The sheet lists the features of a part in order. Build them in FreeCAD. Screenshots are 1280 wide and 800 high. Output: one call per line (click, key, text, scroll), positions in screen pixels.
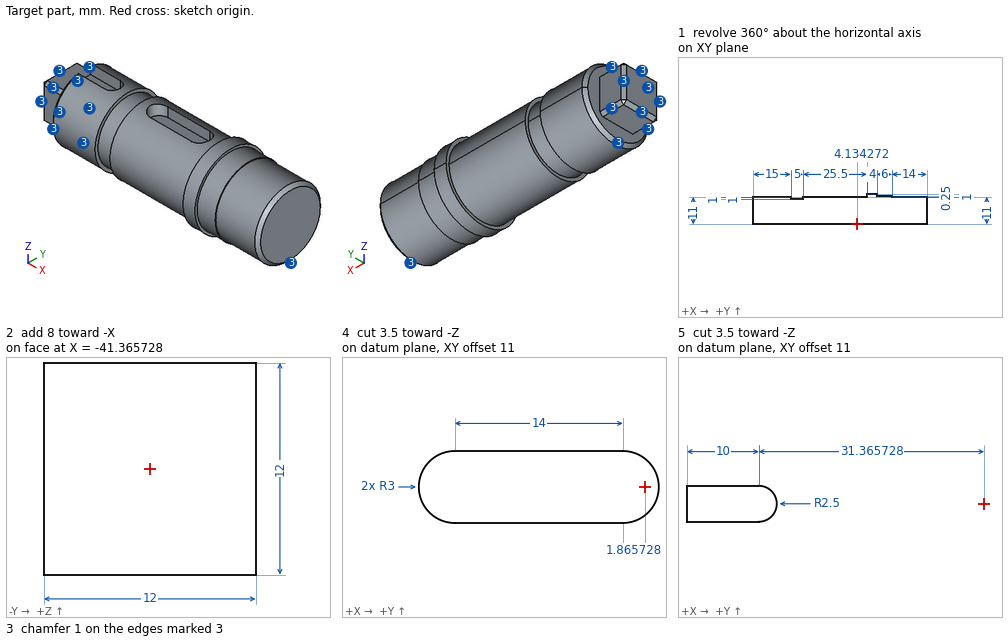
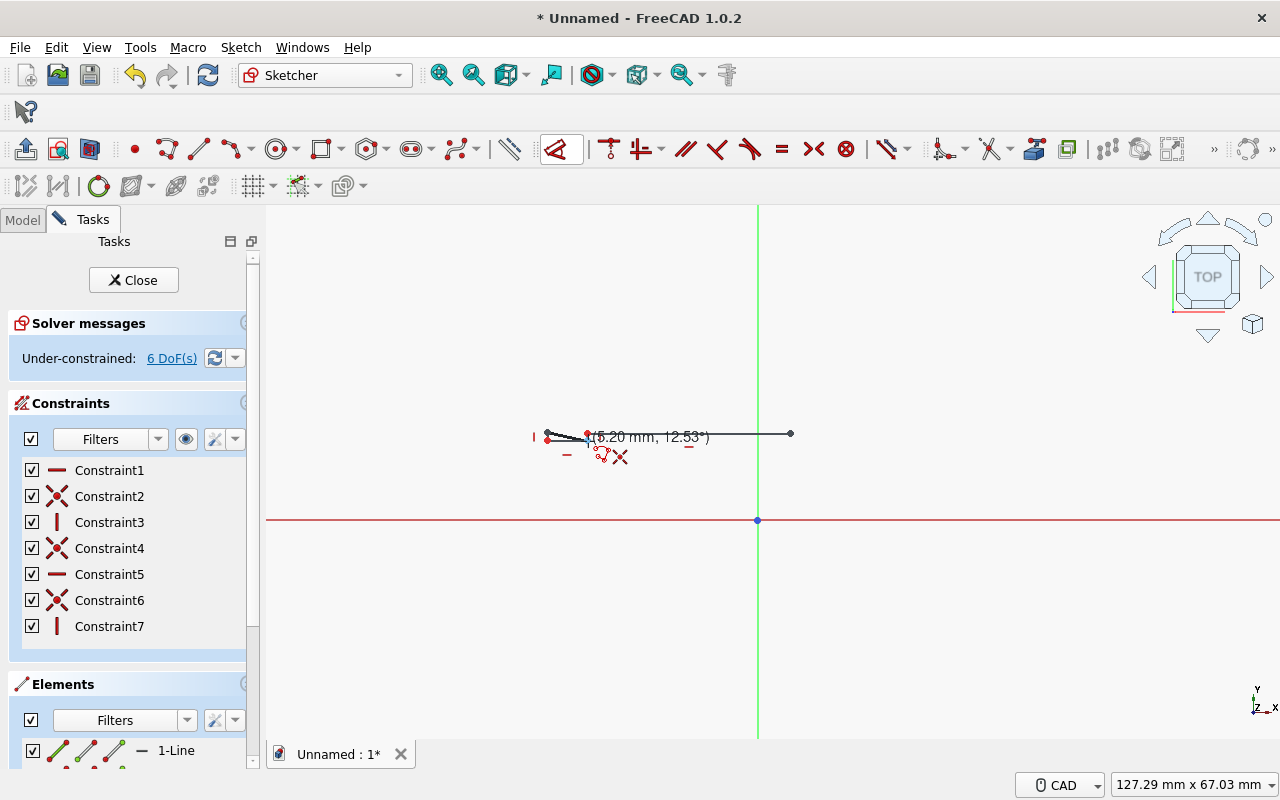
click(428, 432)
click(428, 520)
click(982, 511)
click(982, 432)
click(870, 432)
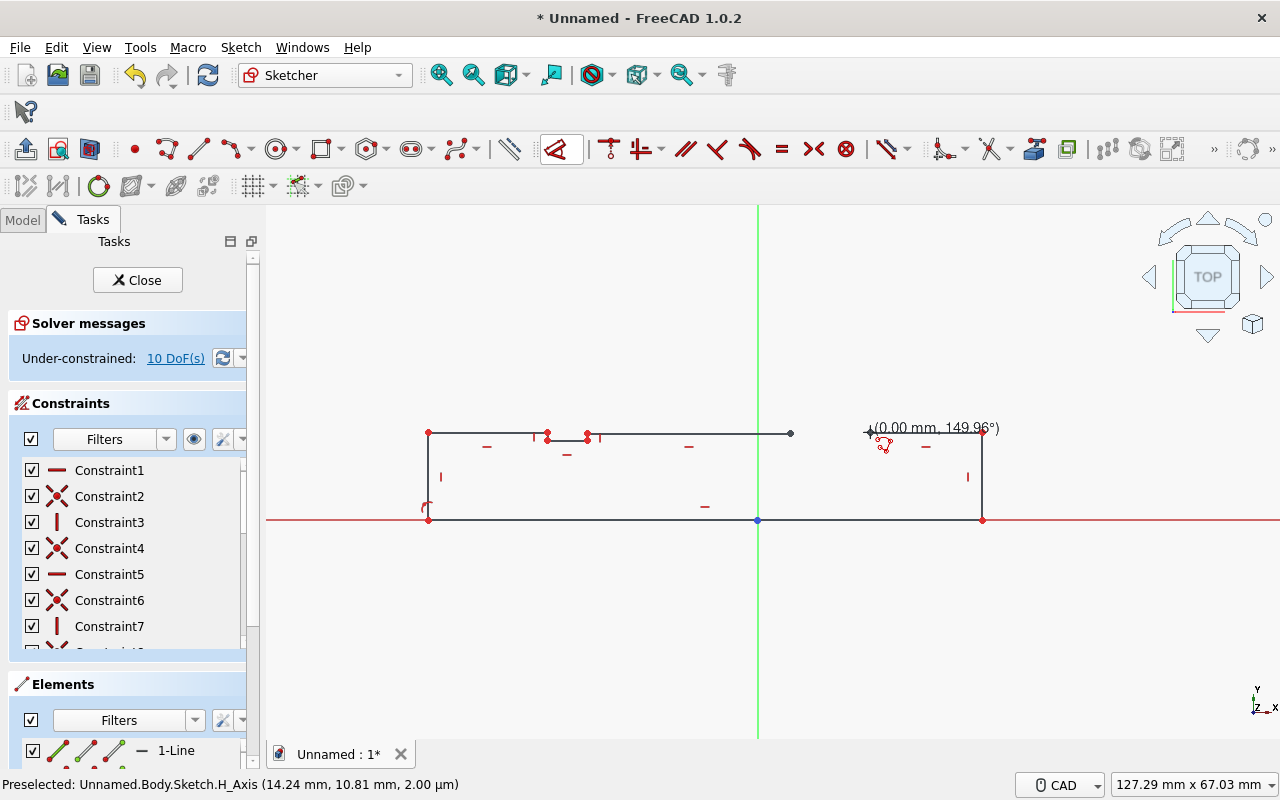
scroll(870, 430, up, 11)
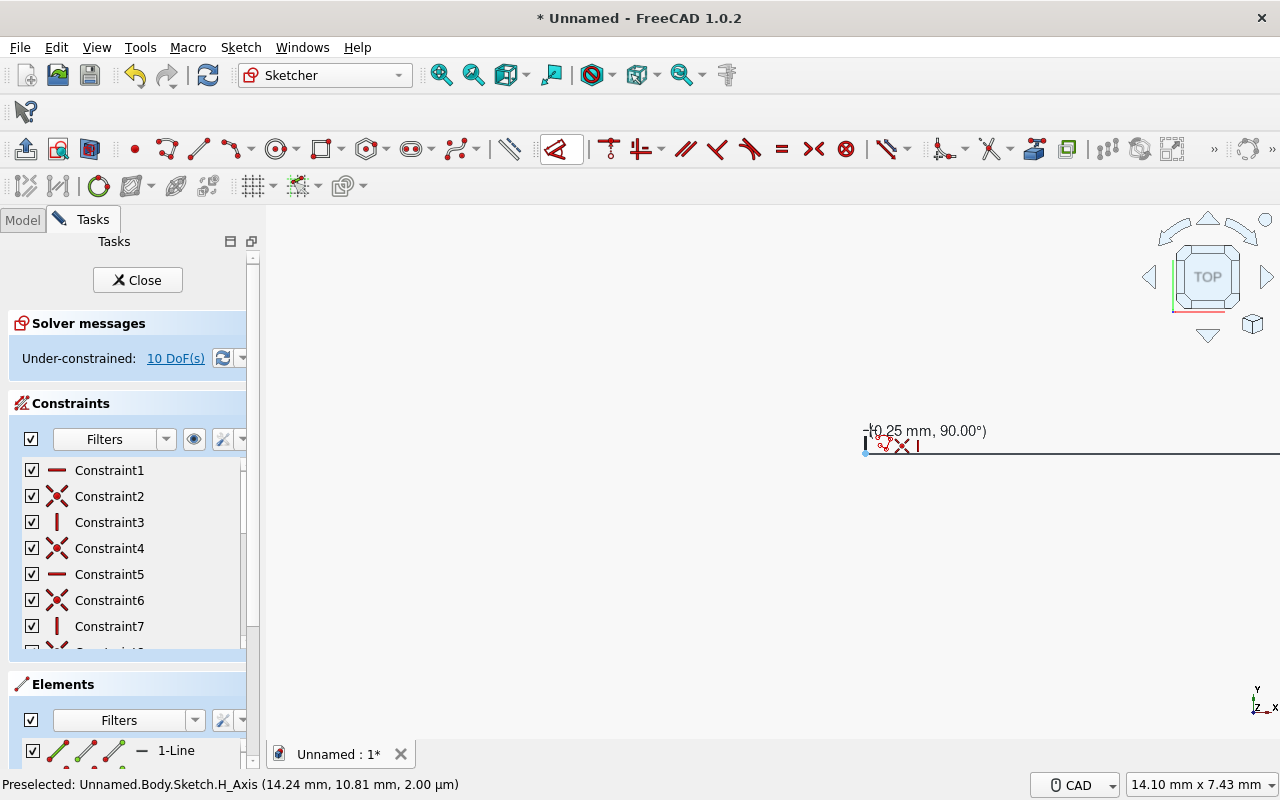
click(865, 431)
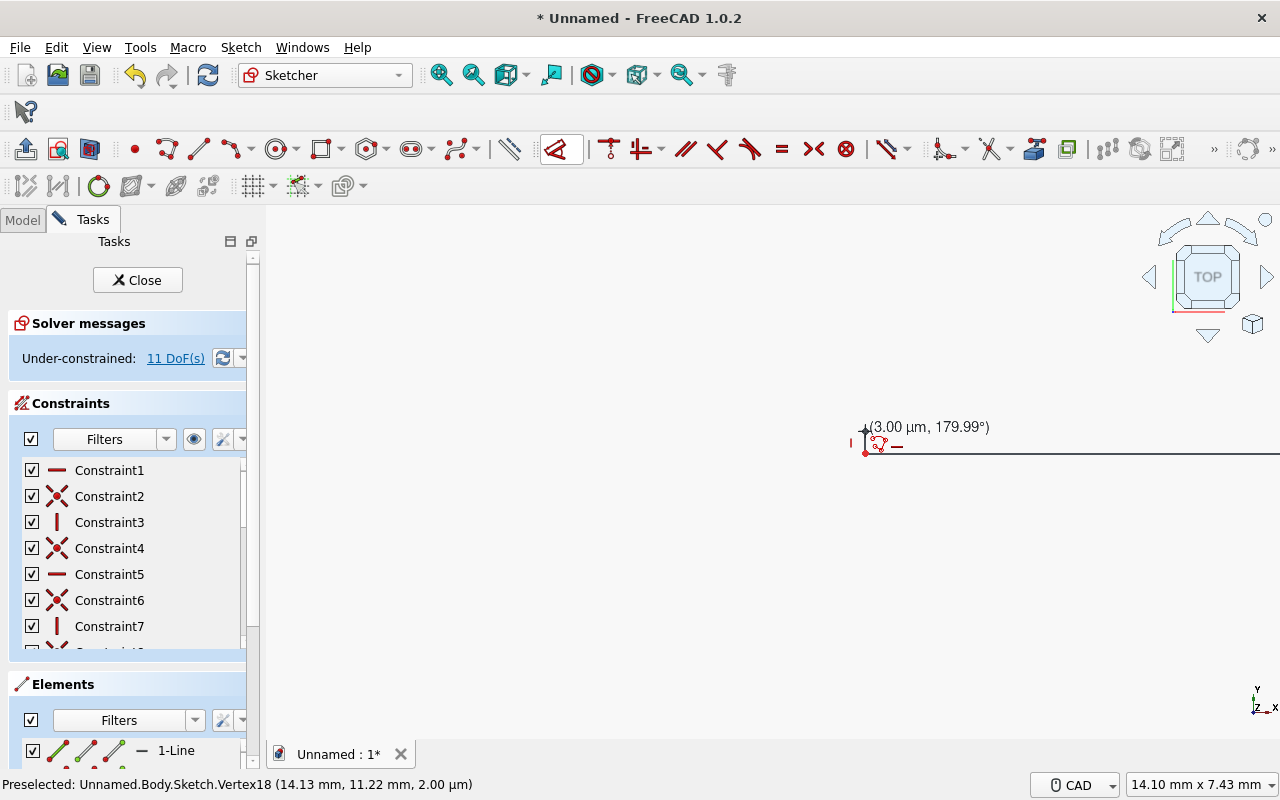
scroll(870, 430, down, 11)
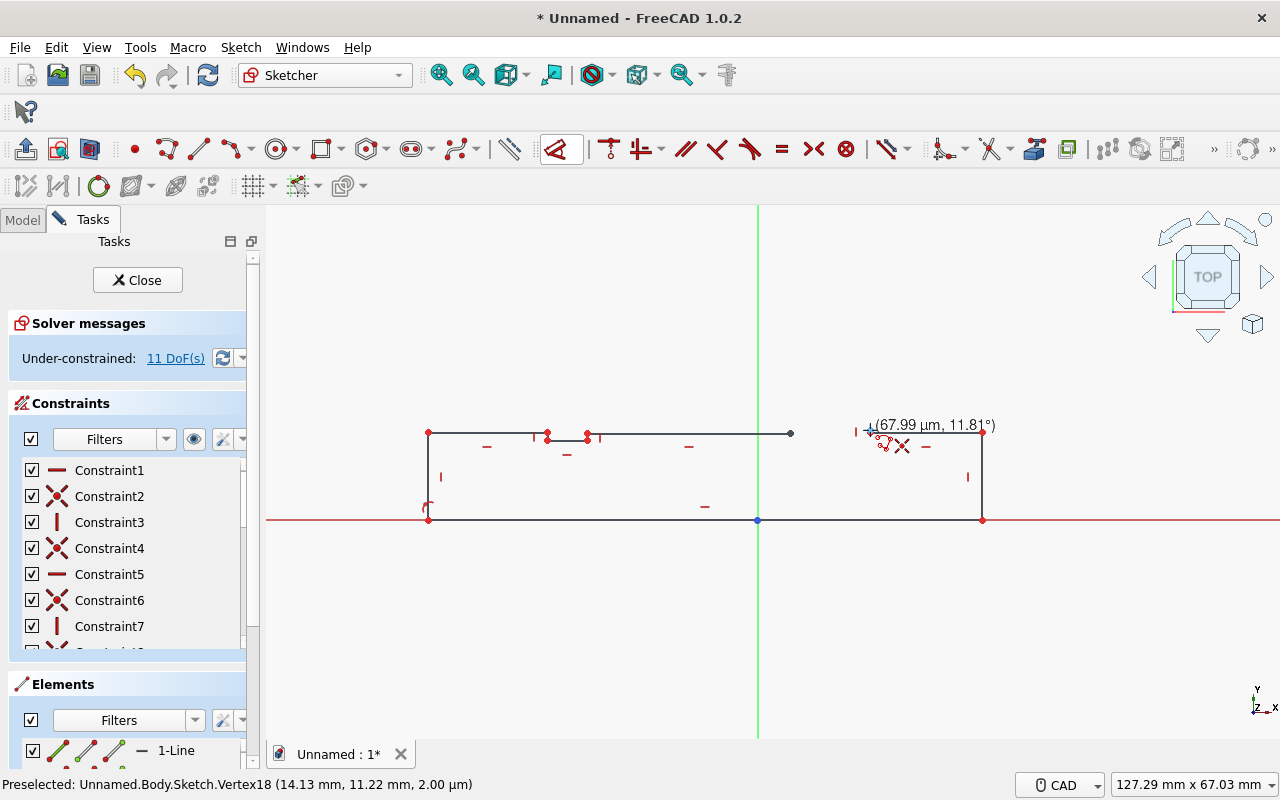
click(822, 430)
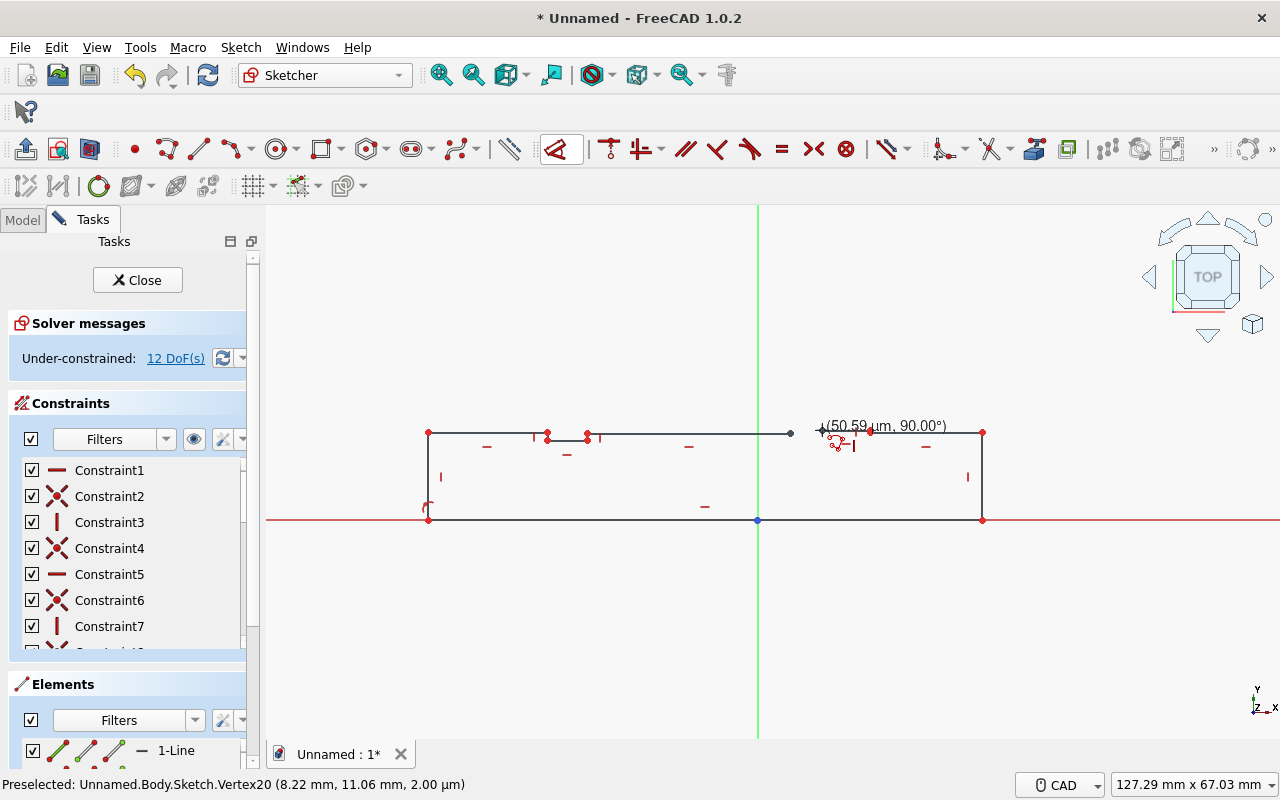
scroll(822, 425, up, 5)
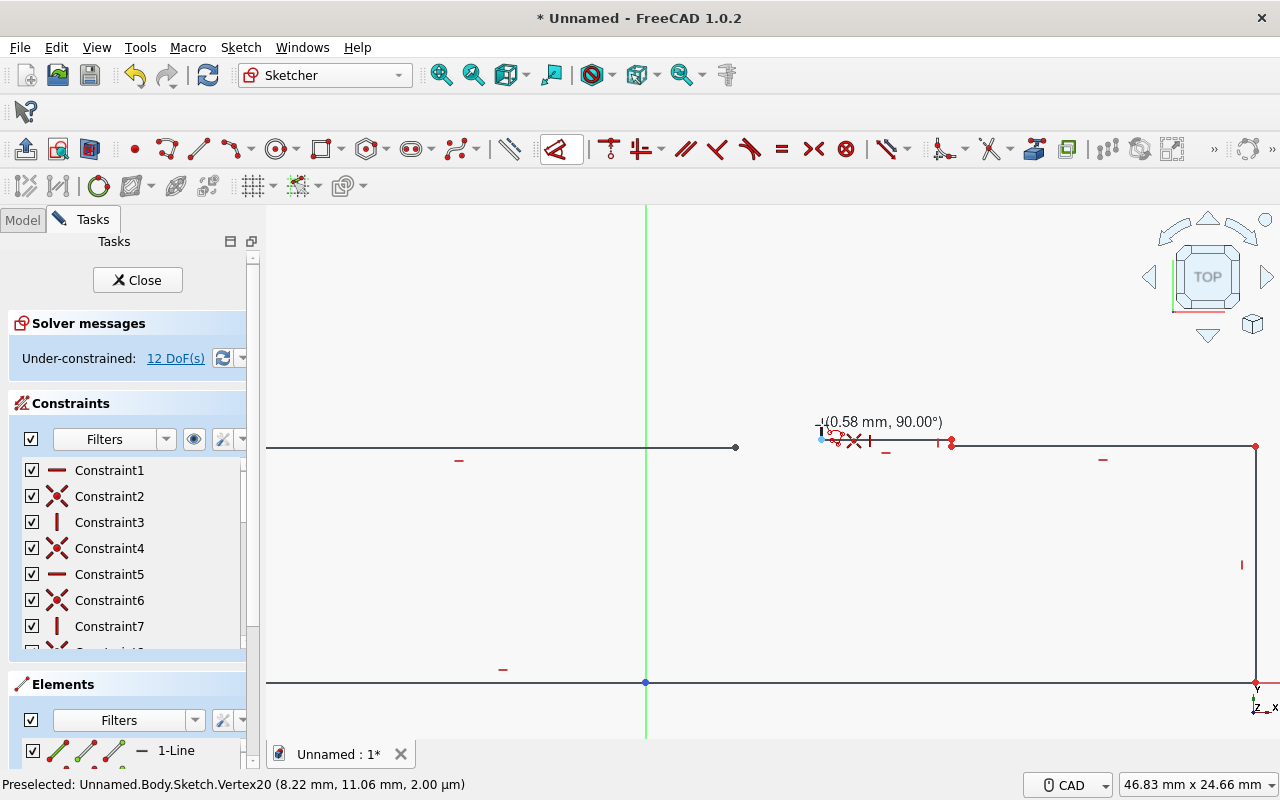
click(821, 423)
click(735, 423)
click(736, 448)
key(Escape)
key(Escape)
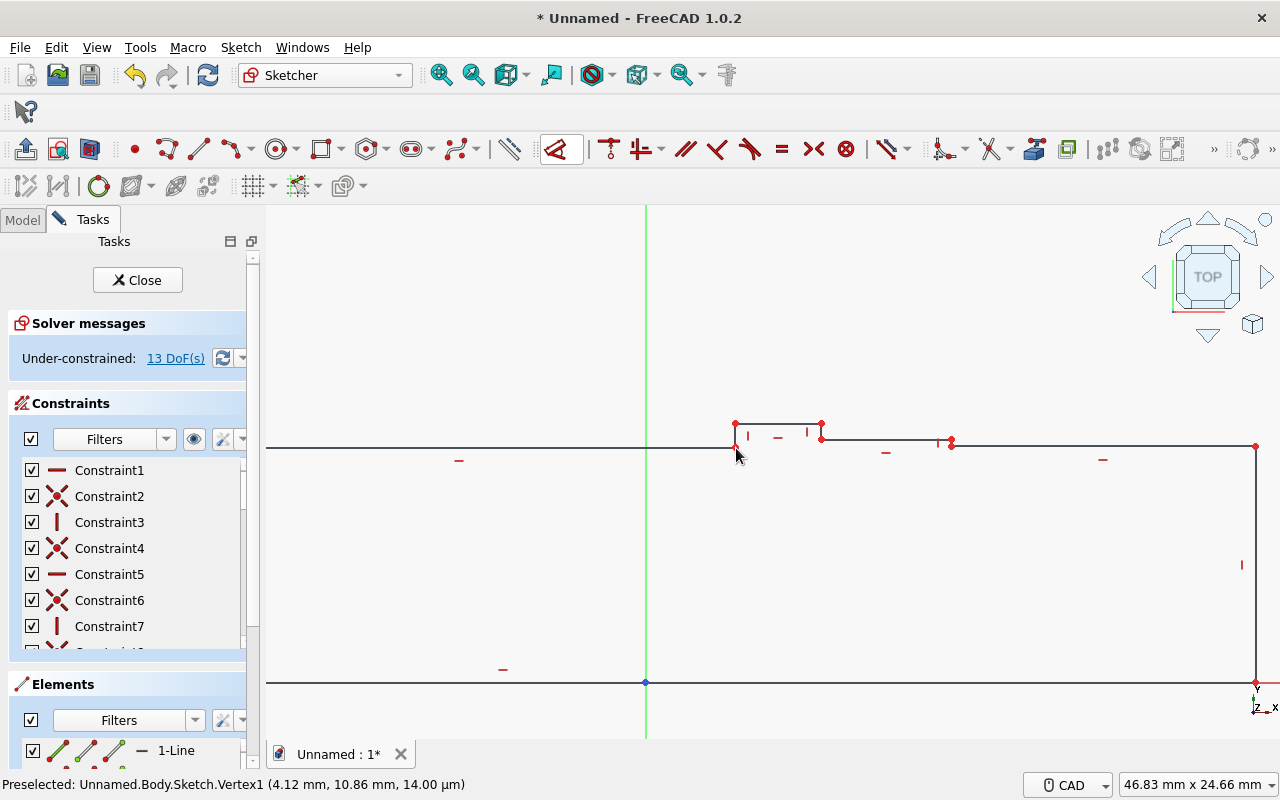
click(556, 150)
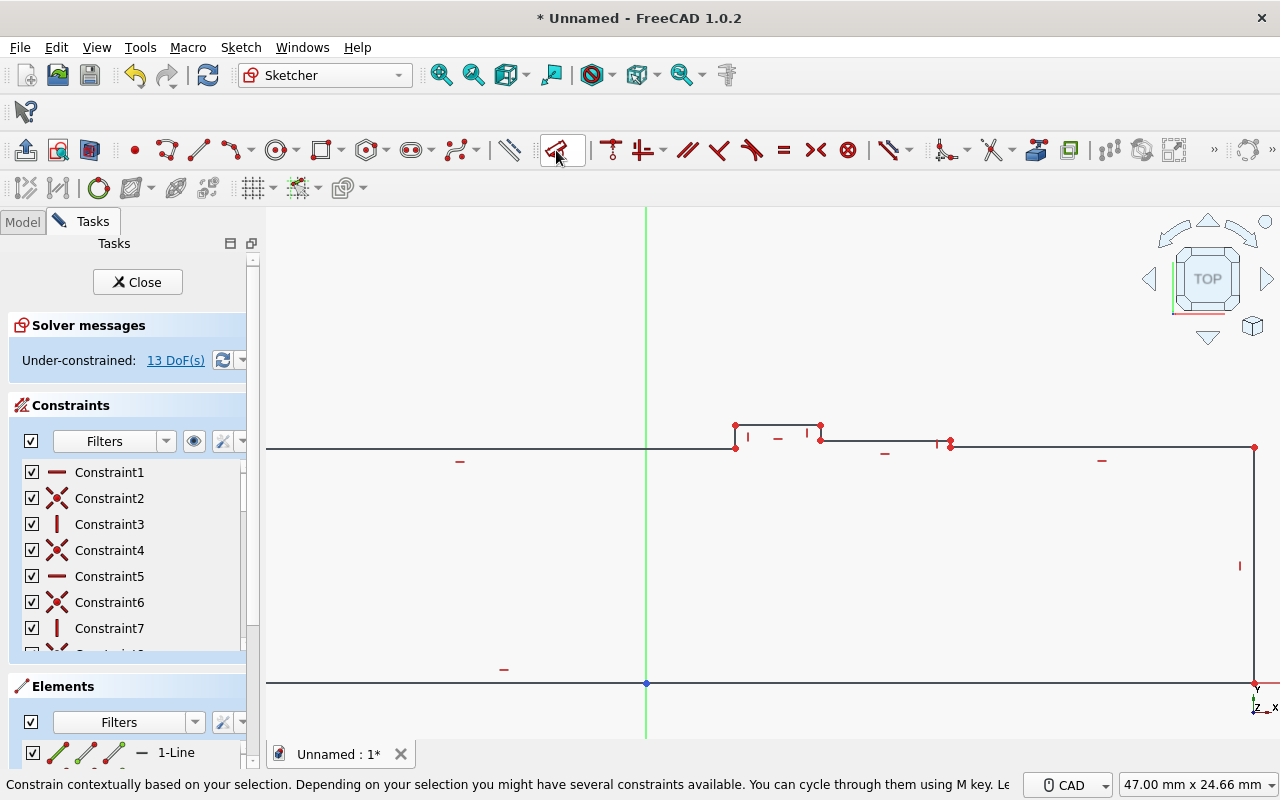
scroll(821, 426, down, 5)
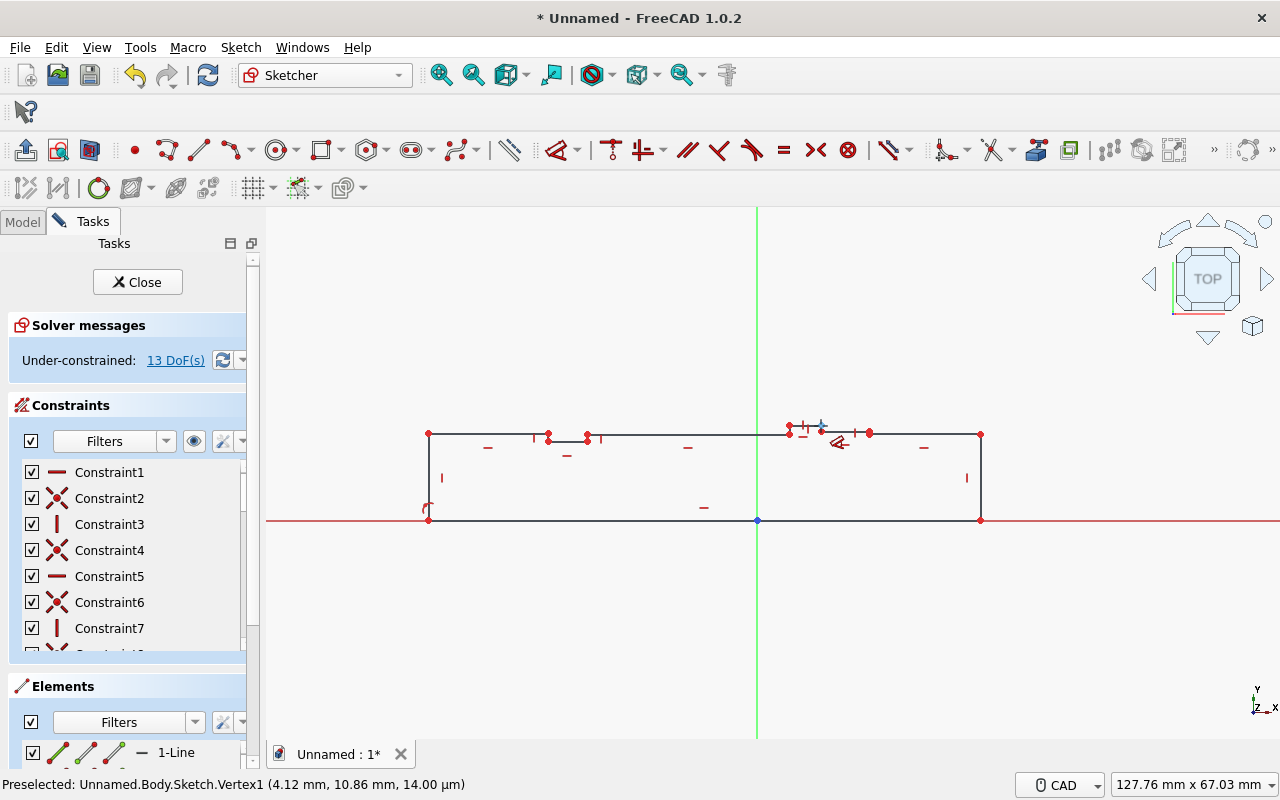
scroll(588, 438, up, 9)